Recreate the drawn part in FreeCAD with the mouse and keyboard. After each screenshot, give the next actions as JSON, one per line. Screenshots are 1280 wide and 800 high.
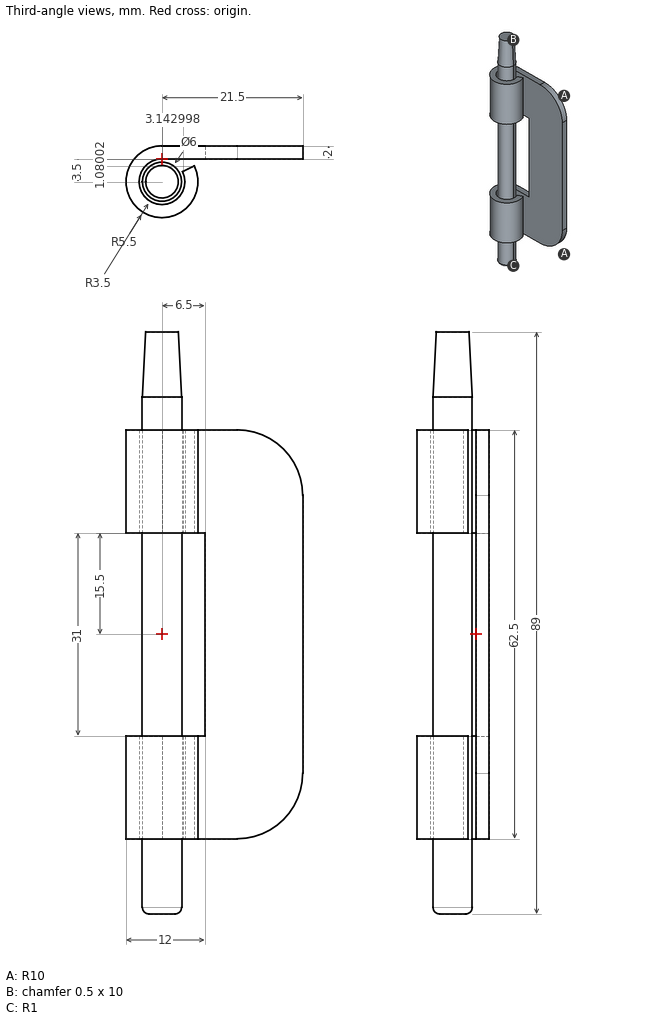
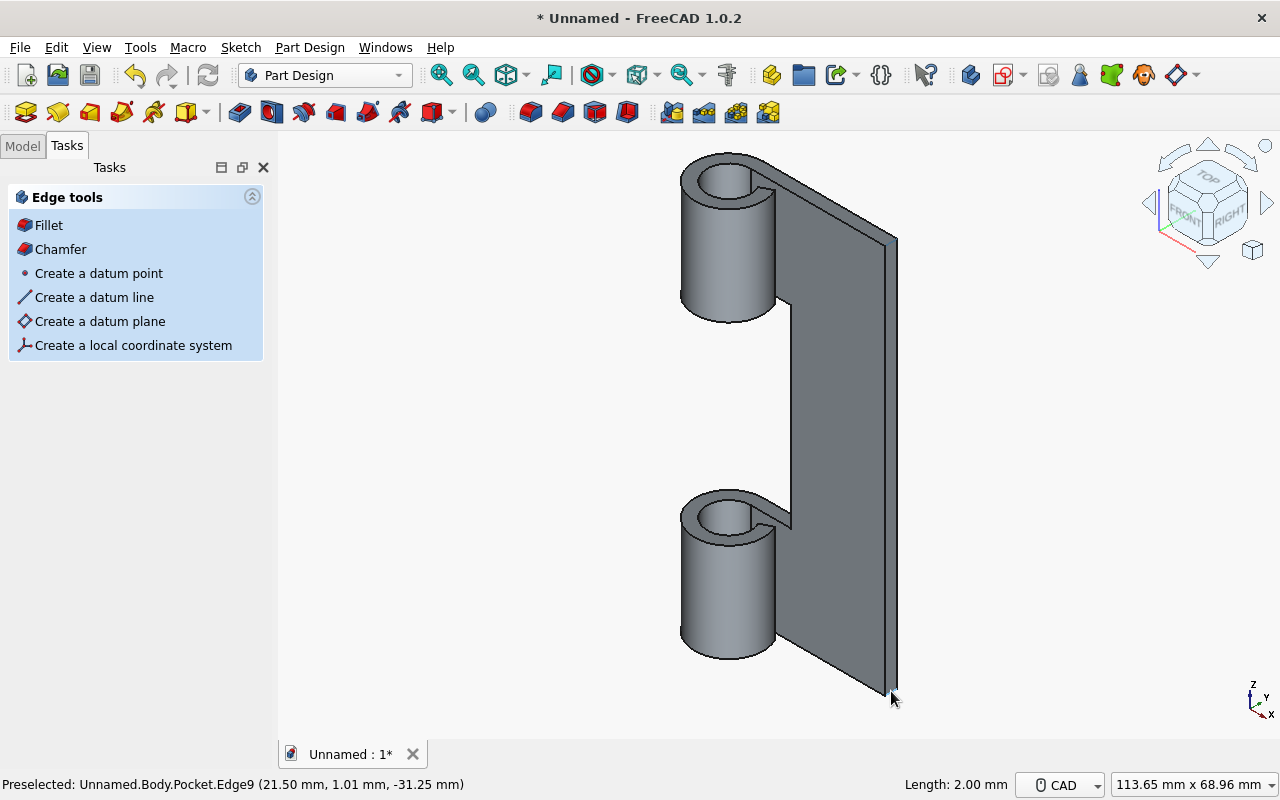
{"action": "key", "text": "2"}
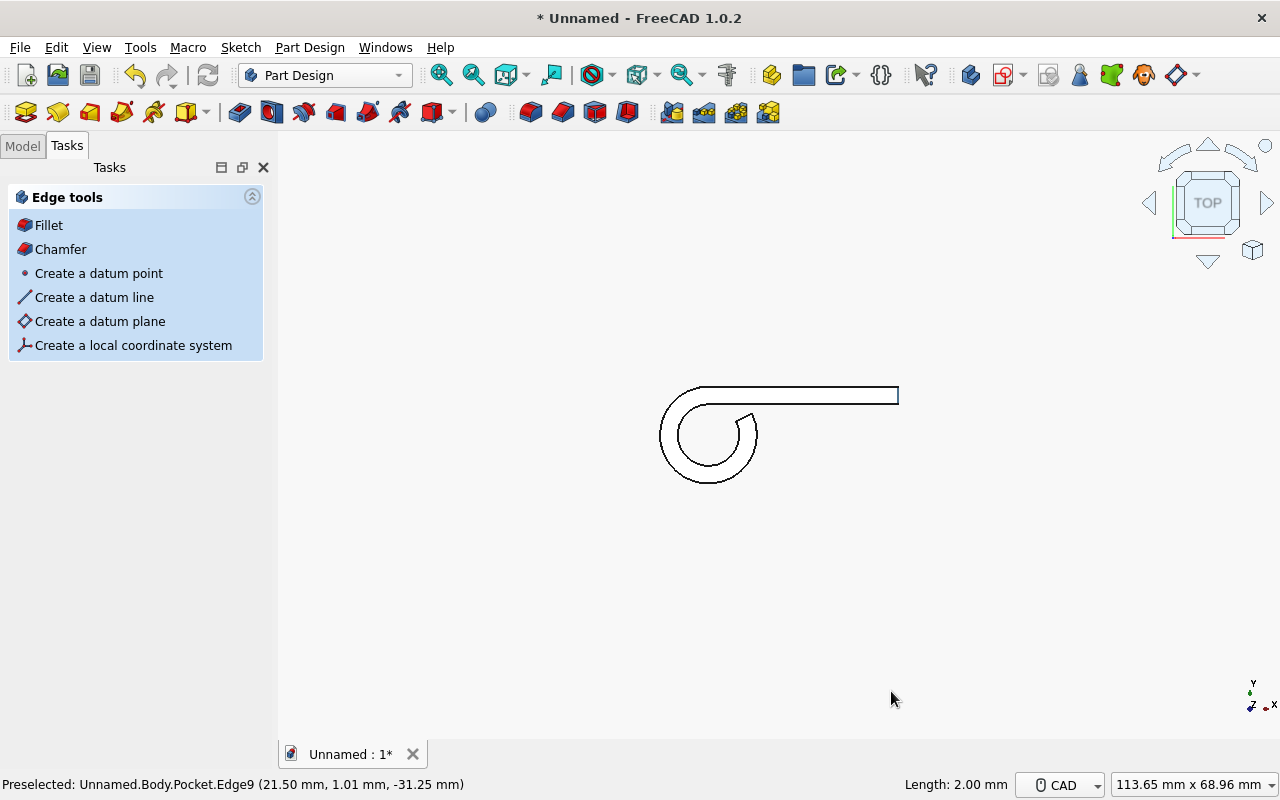
{"action": "key", "text": "v f"}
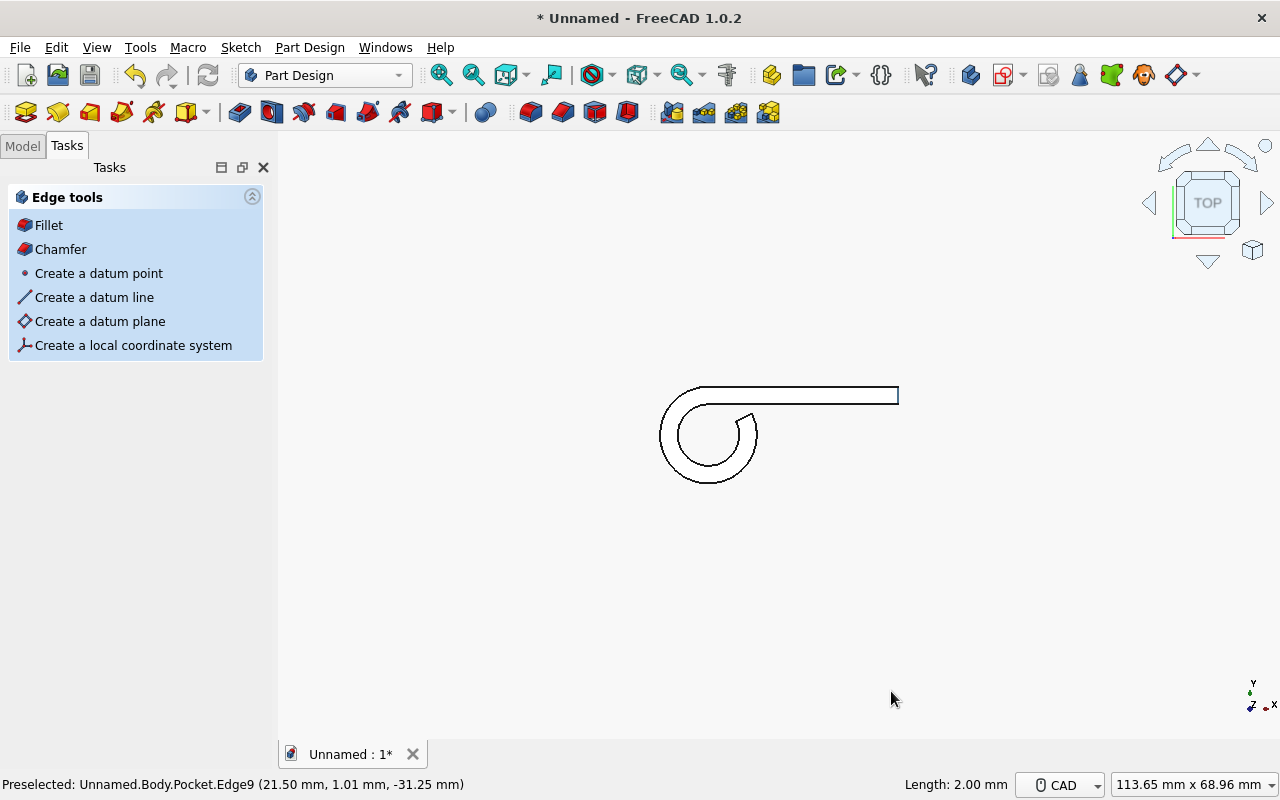
{"action": "scroll", "coordinate": [898, 394], "scroll_direction": "up", "scroll_amount": 5}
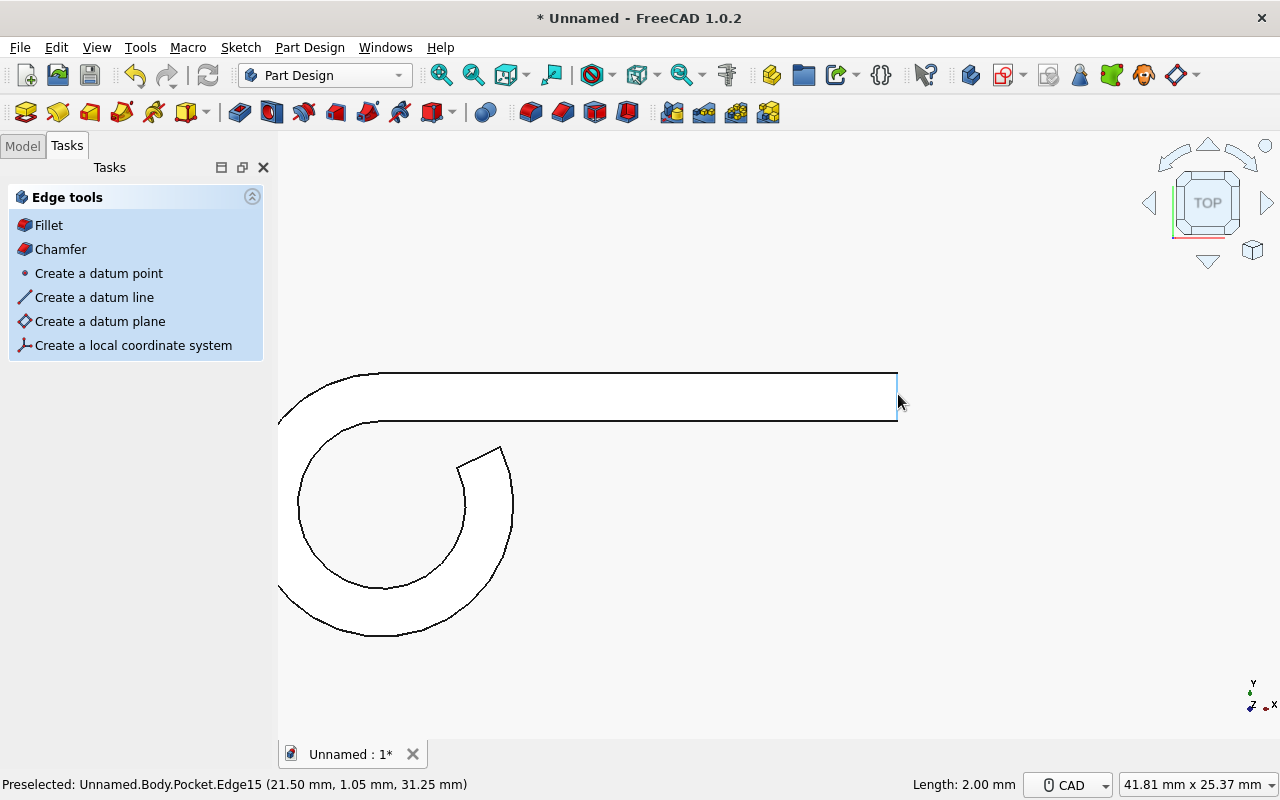
{"action": "key", "text": "v f"}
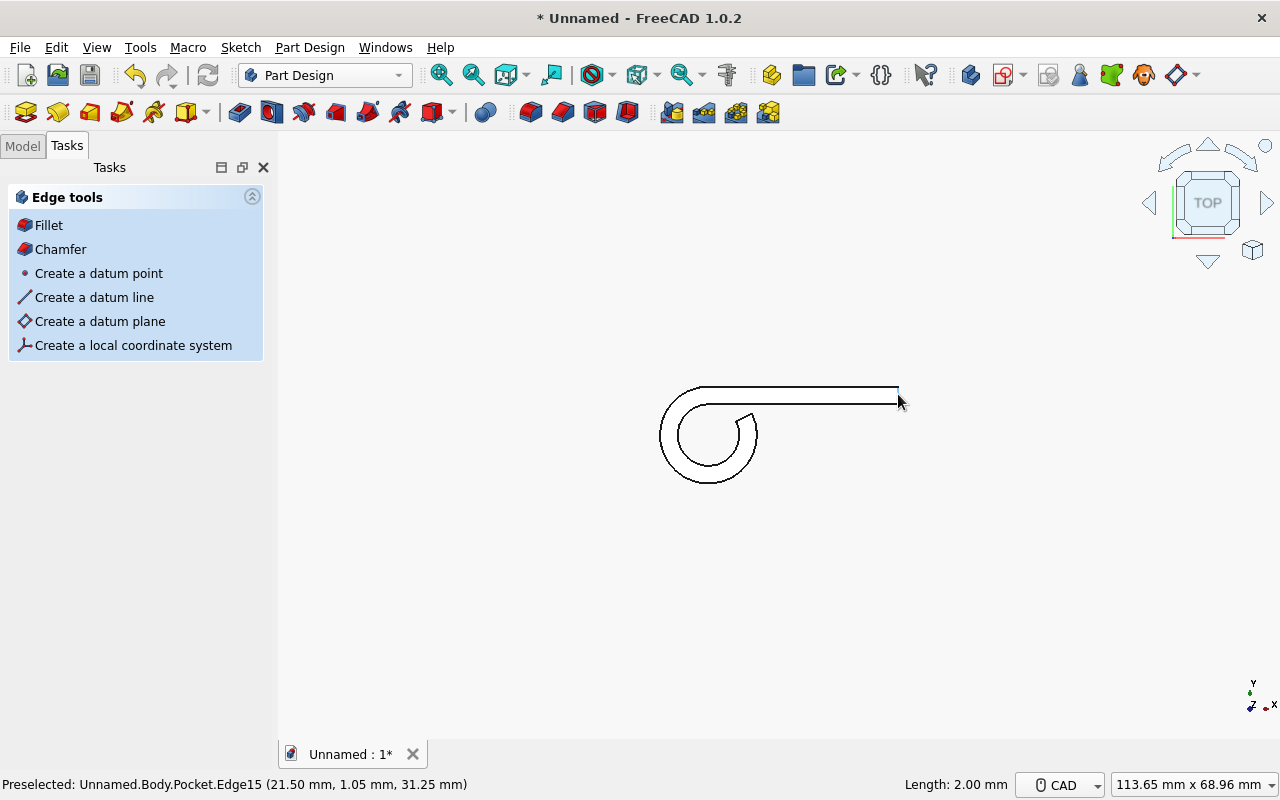
{"action": "key", "text": "1"}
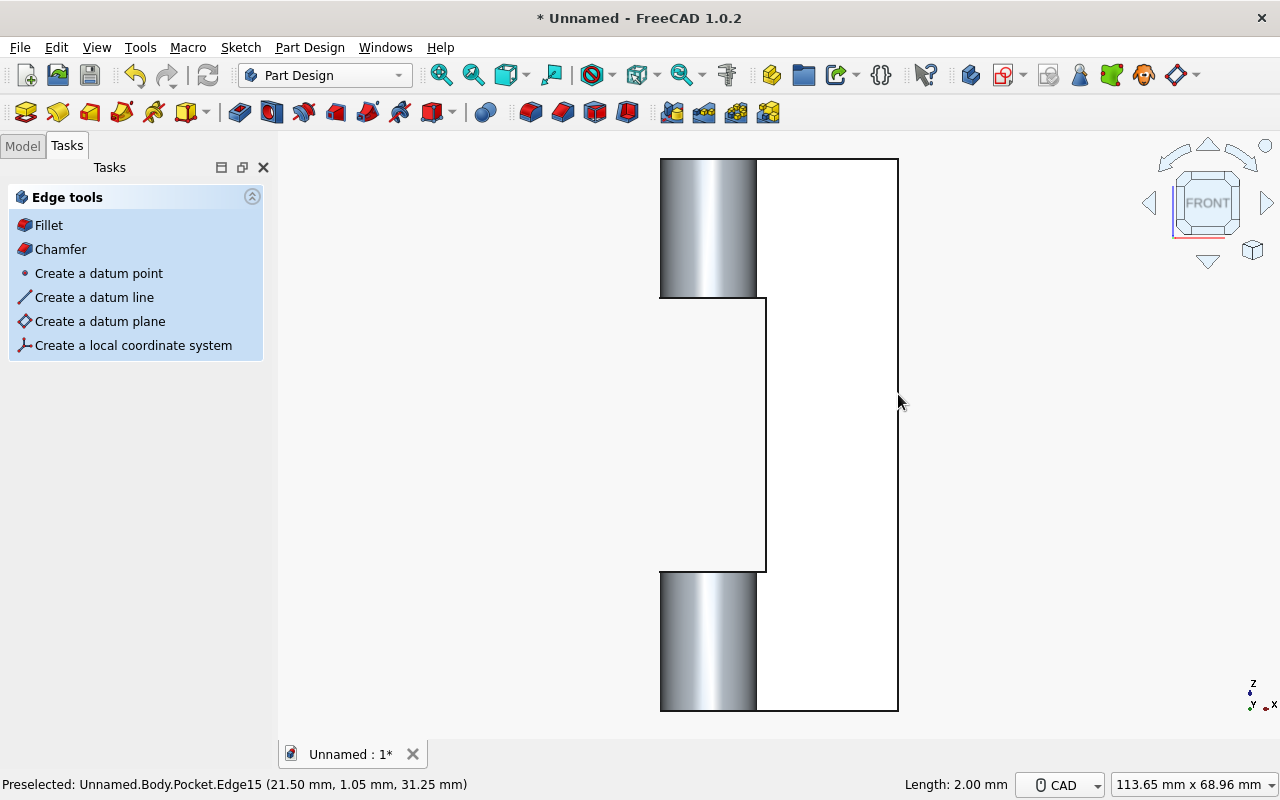
{"action": "scroll", "coordinate": [898, 710], "scroll_direction": "up", "scroll_amount": 5}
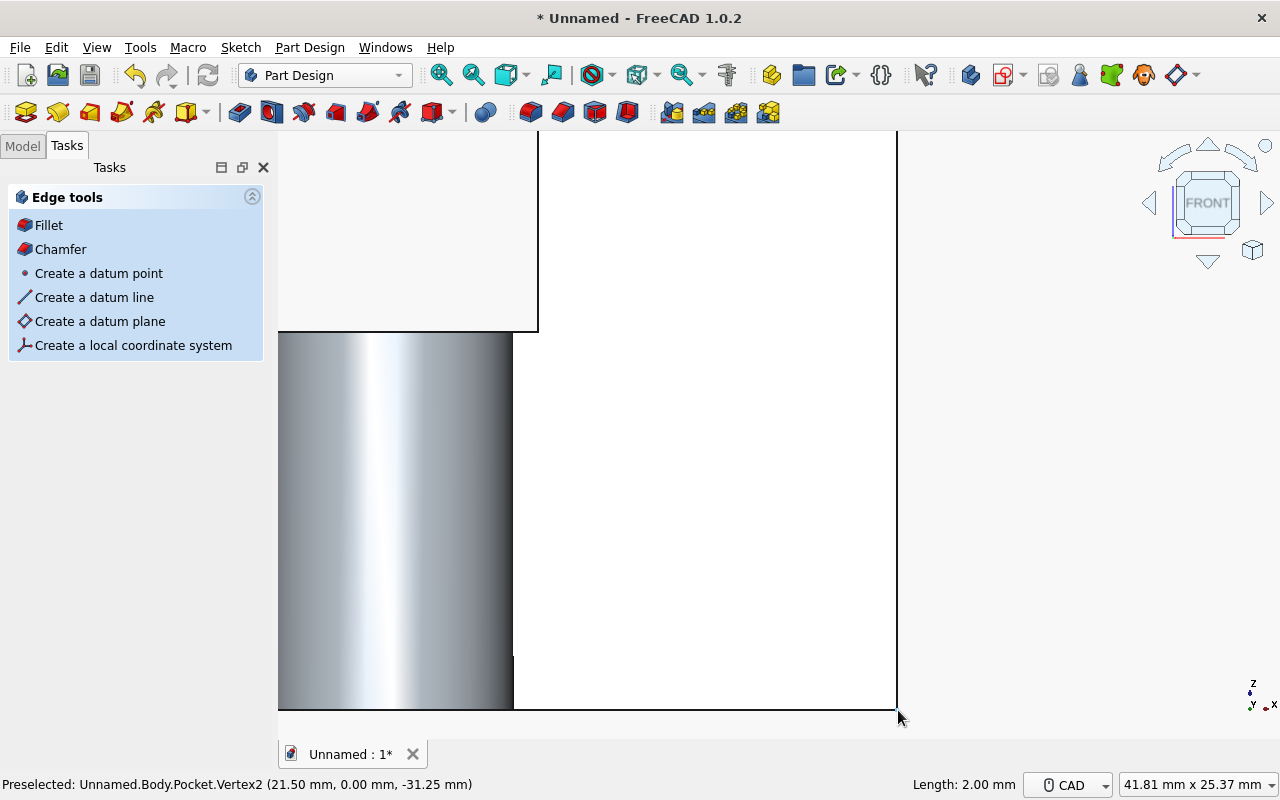
{"action": "left_click", "coordinate": [442, 76]}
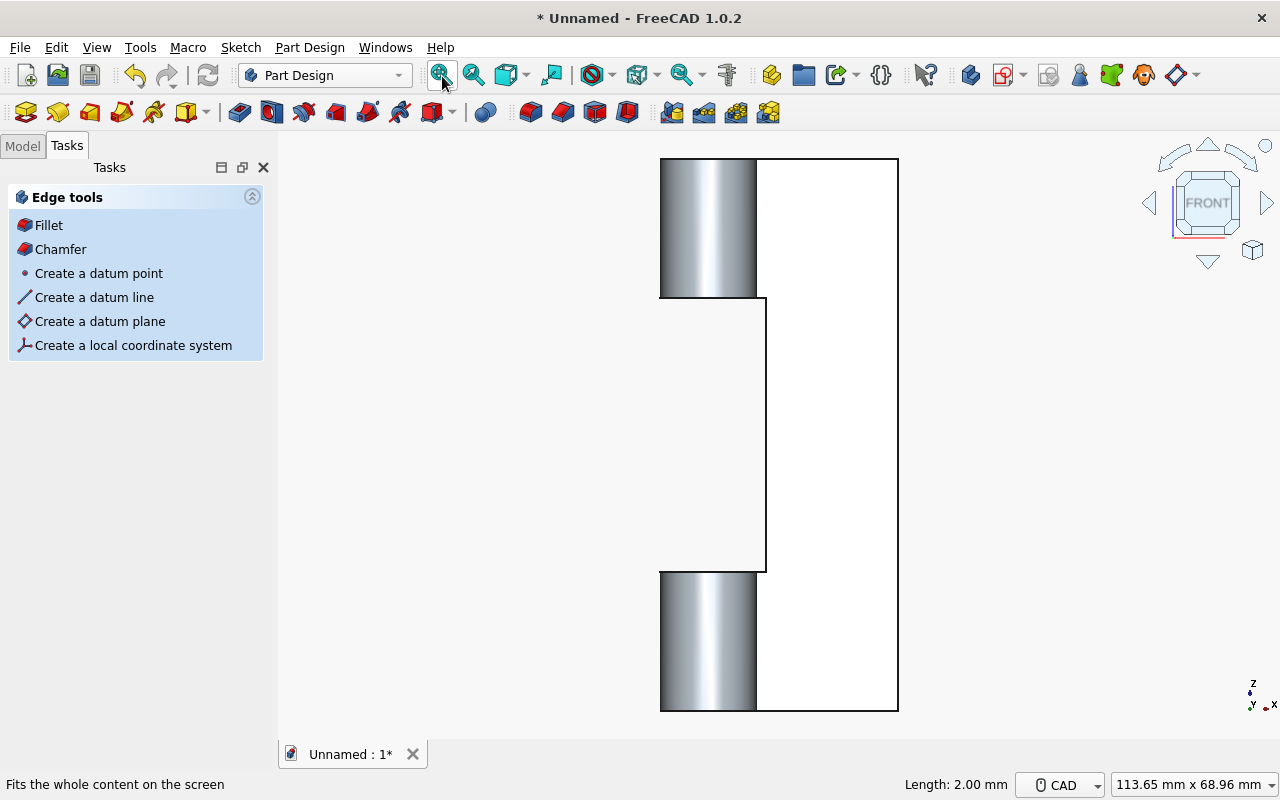
{"action": "key", "text": "3"}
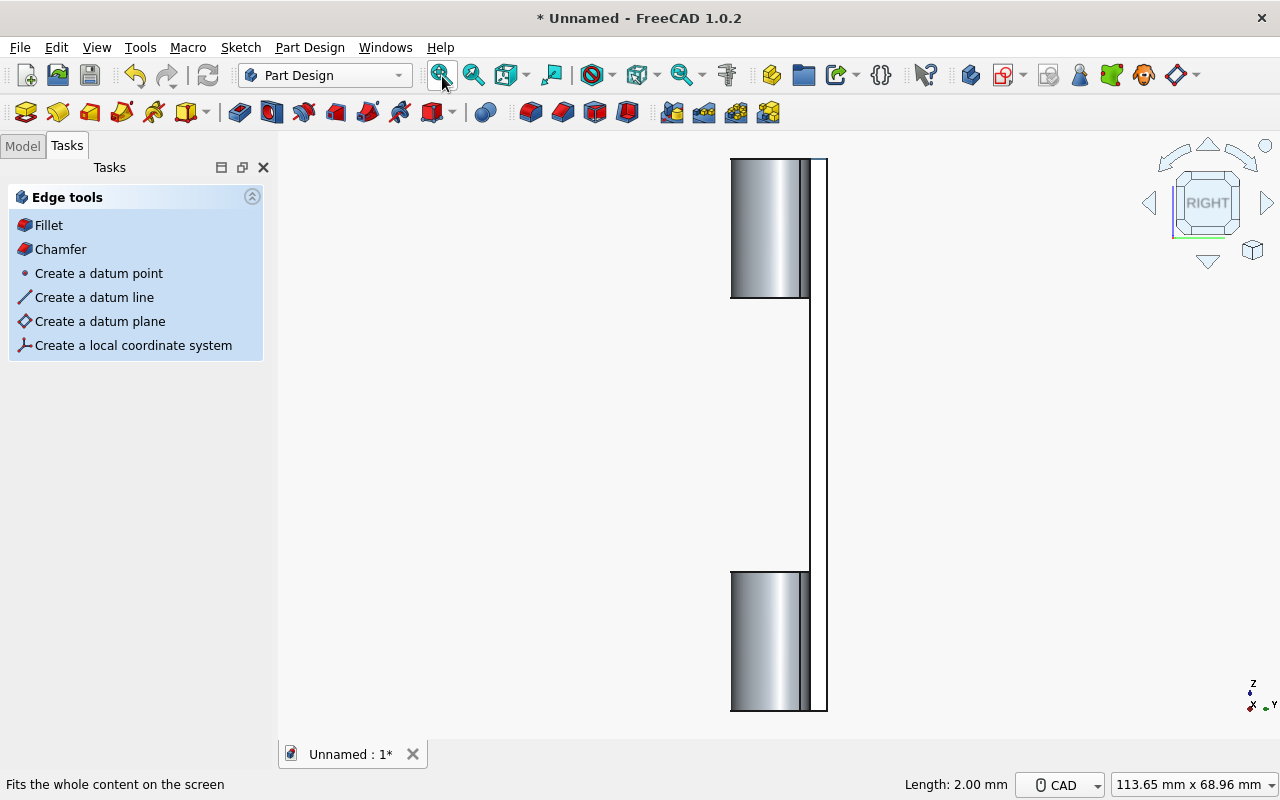
{"action": "left_click", "coordinate": [819, 710], "text": "ctrl"}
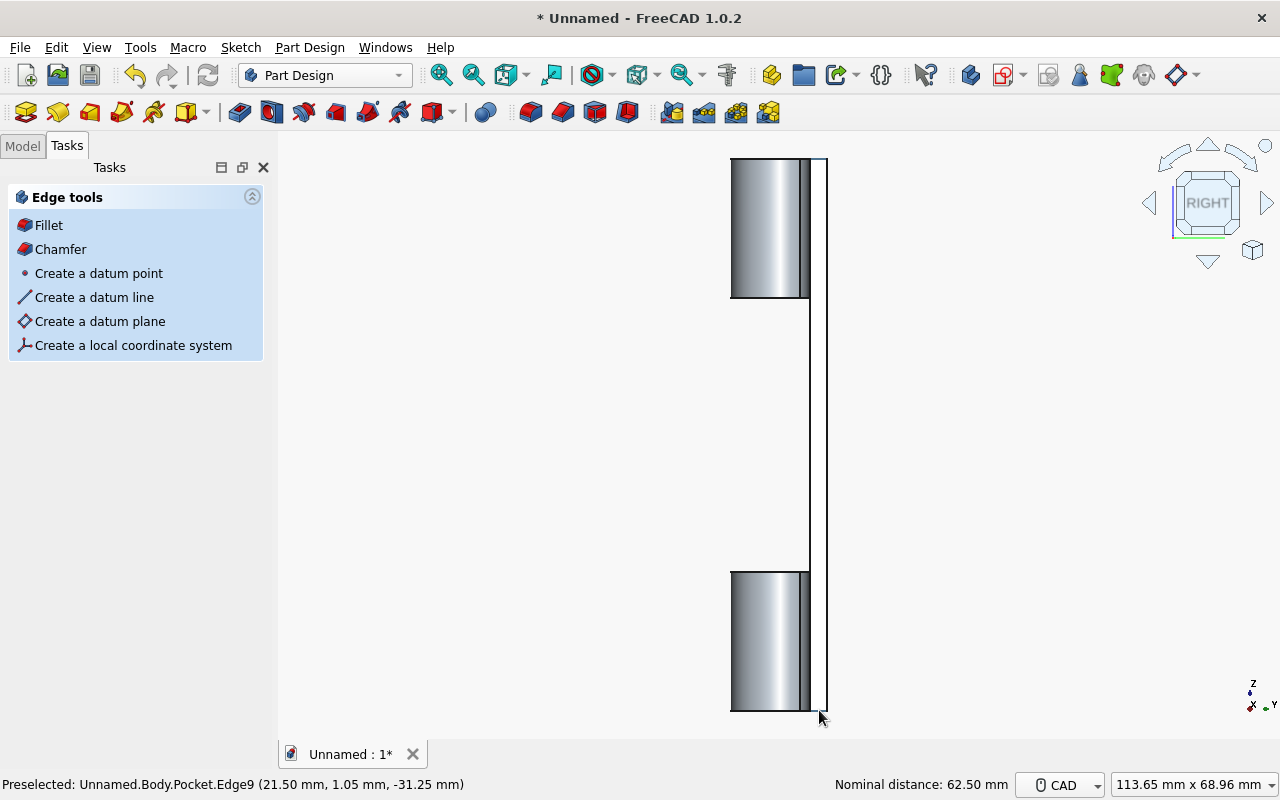
{"action": "left_click", "coordinate": [532, 112]}